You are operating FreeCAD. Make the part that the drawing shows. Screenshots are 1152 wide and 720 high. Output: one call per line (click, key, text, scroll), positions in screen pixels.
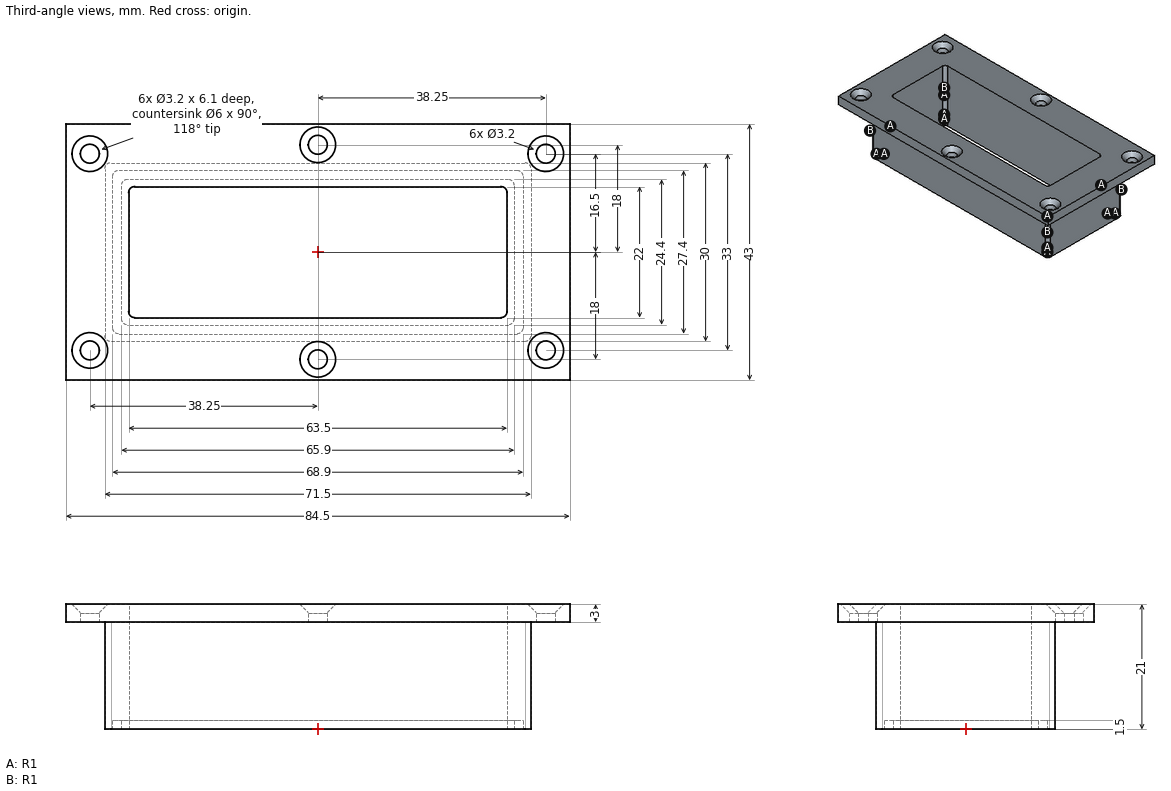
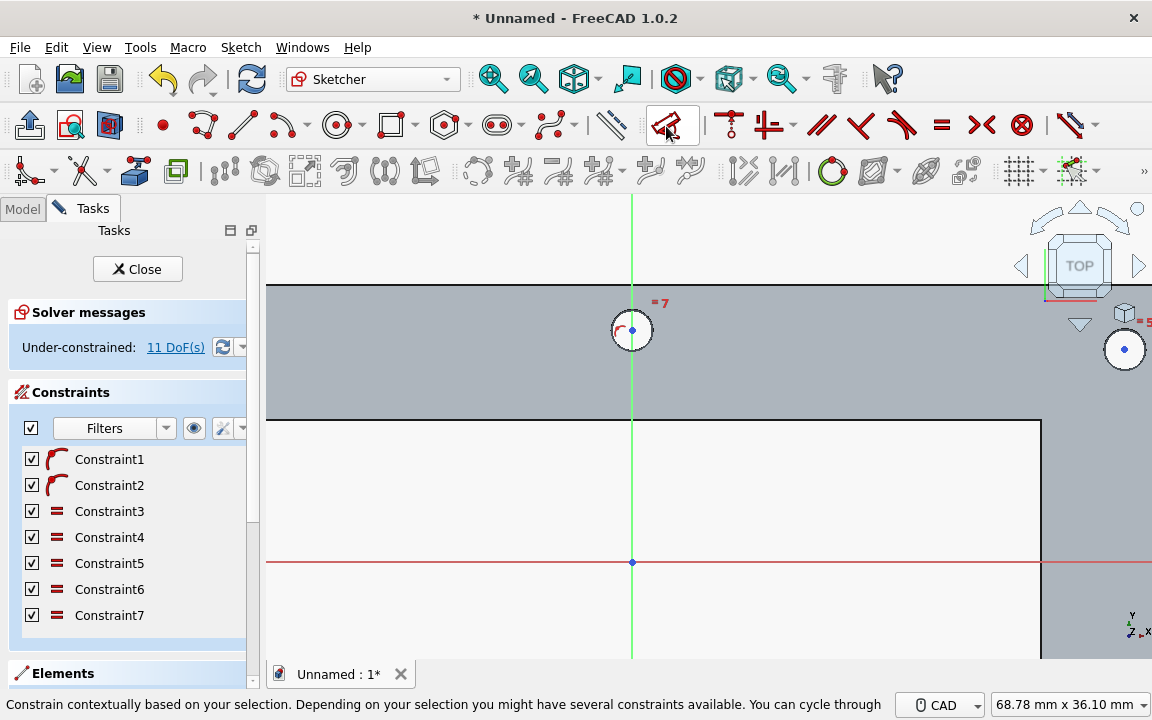
scroll(647, 316, down, 4)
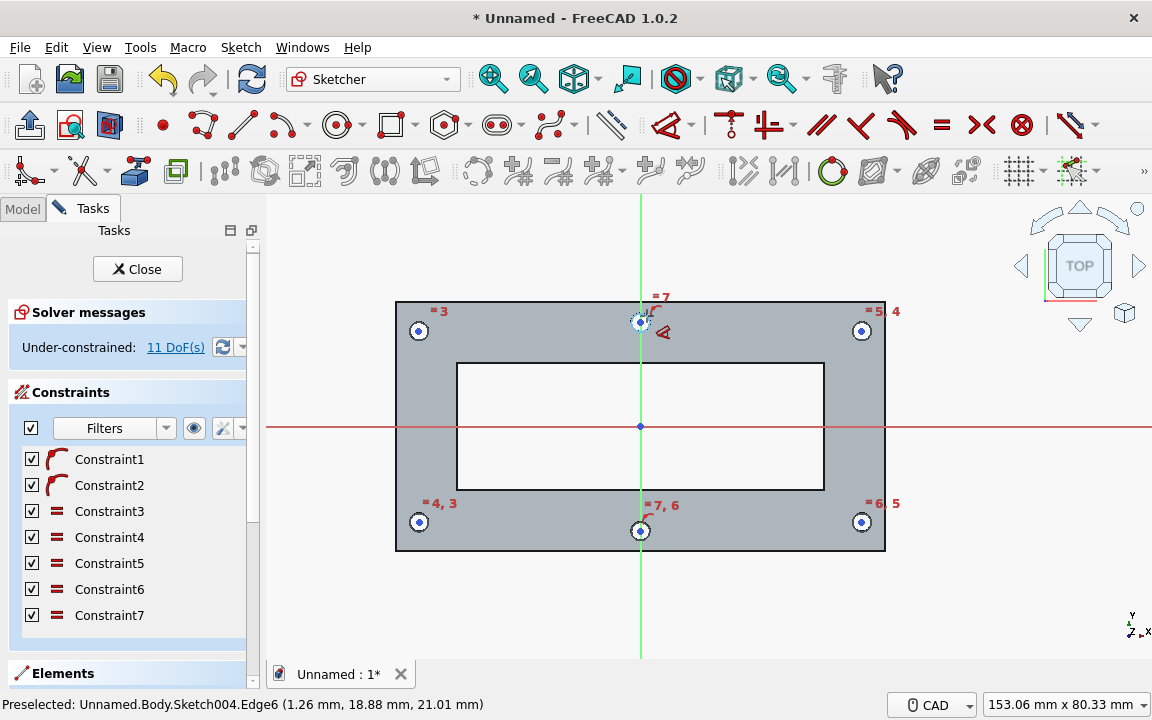
scroll(425, 325, up, 4)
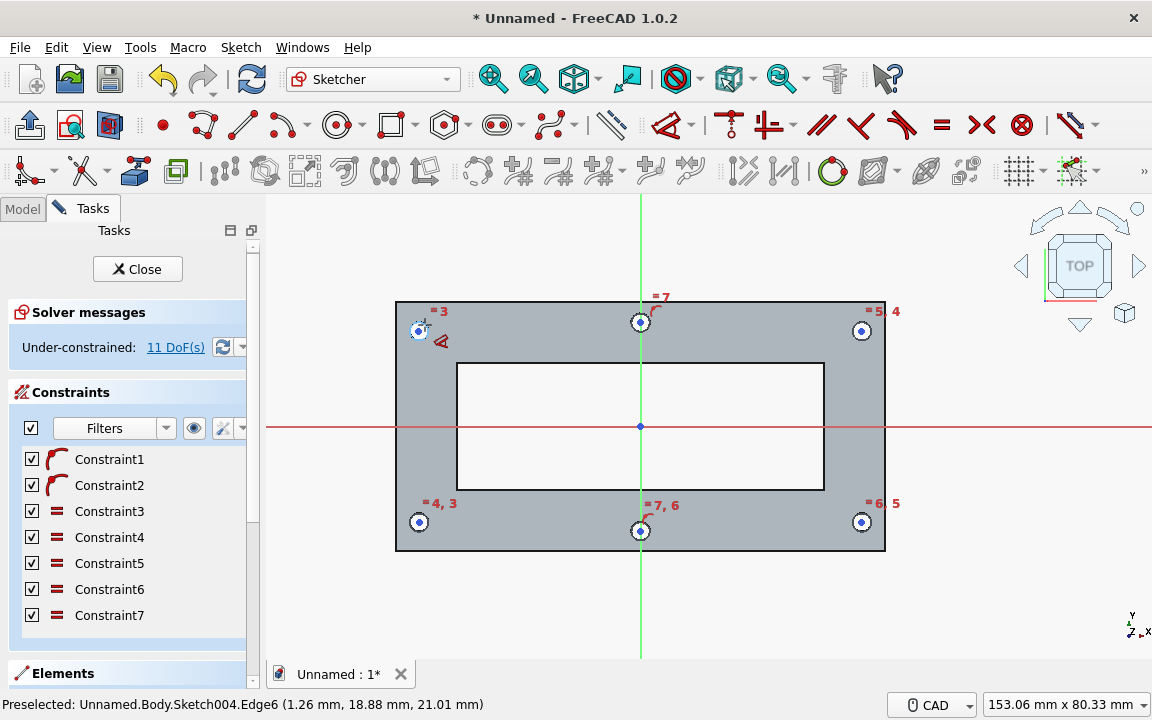
click(426, 325)
click(449, 303)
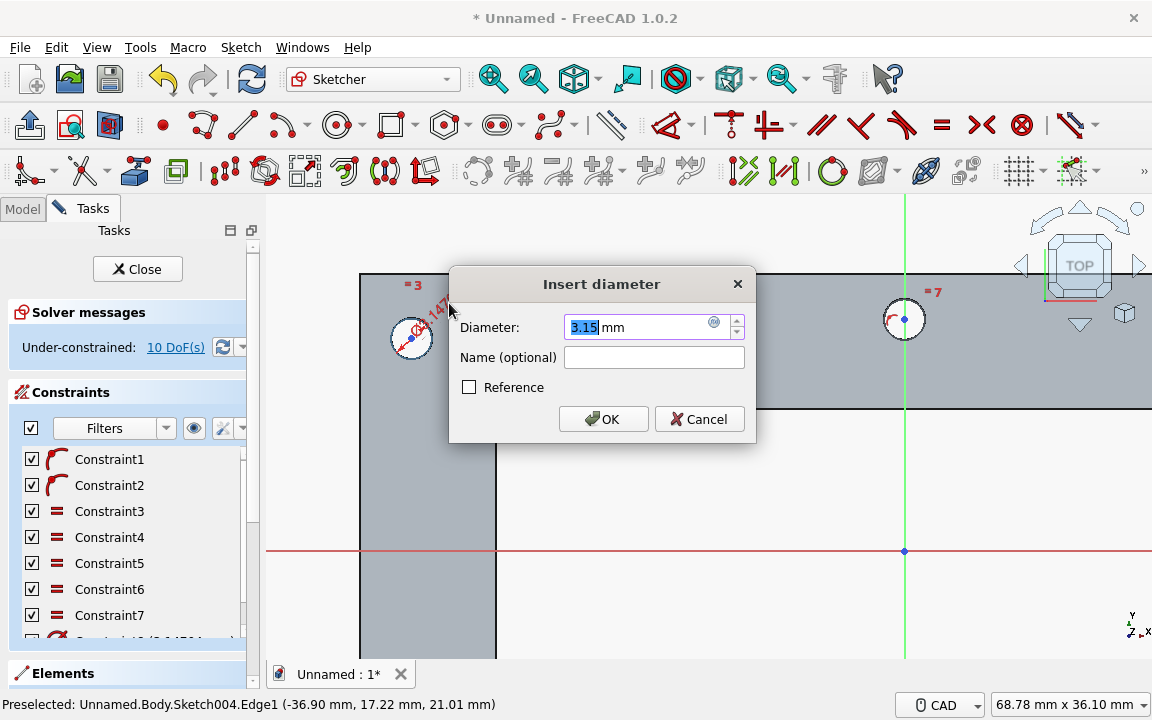
text(3.2)
key(Return)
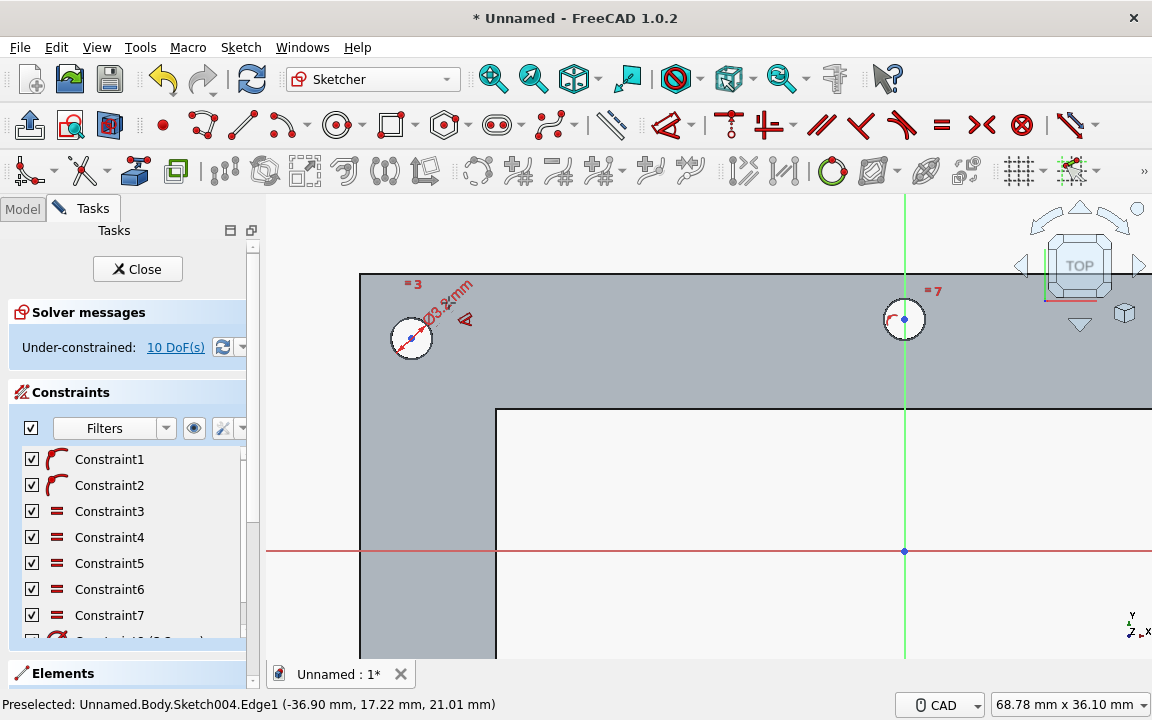
scroll(425, 325, down, 4)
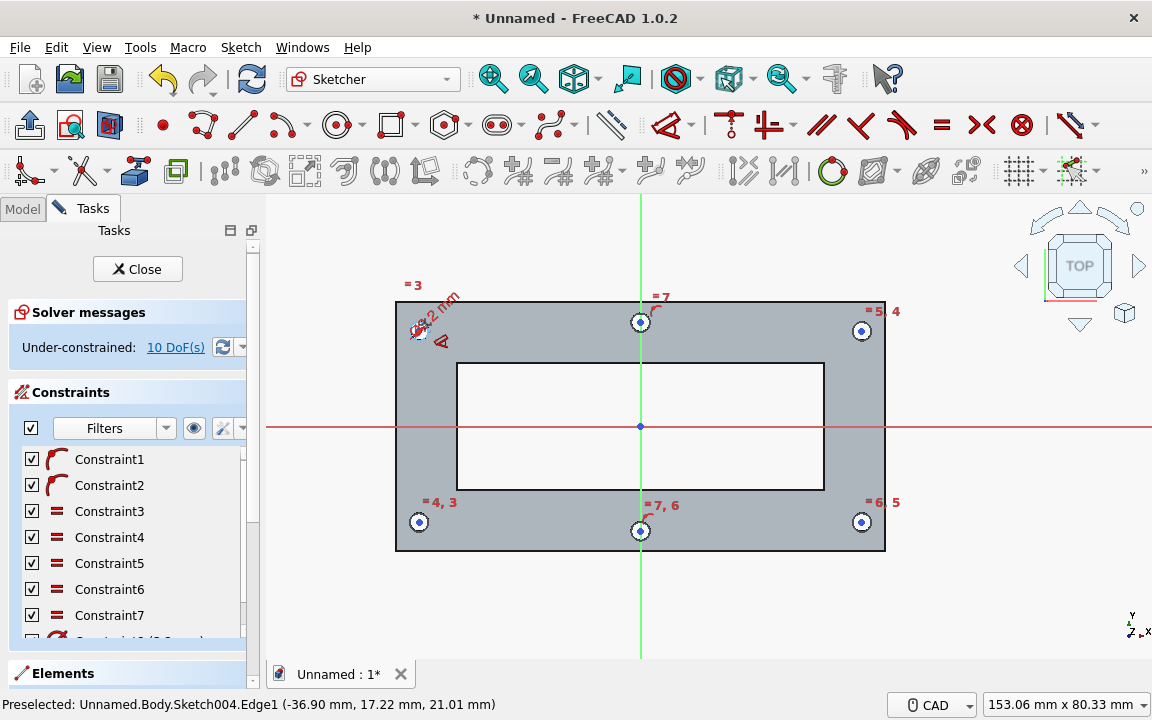
click(641, 531)
click(675, 479)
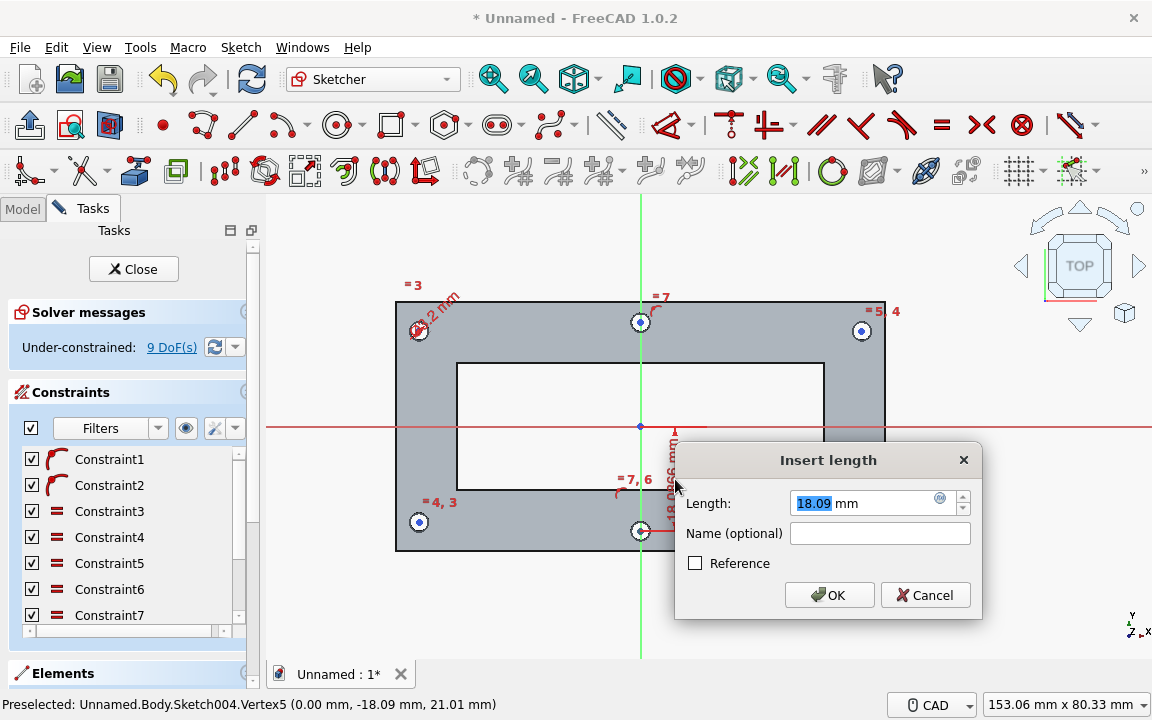
text(18)
key(Return)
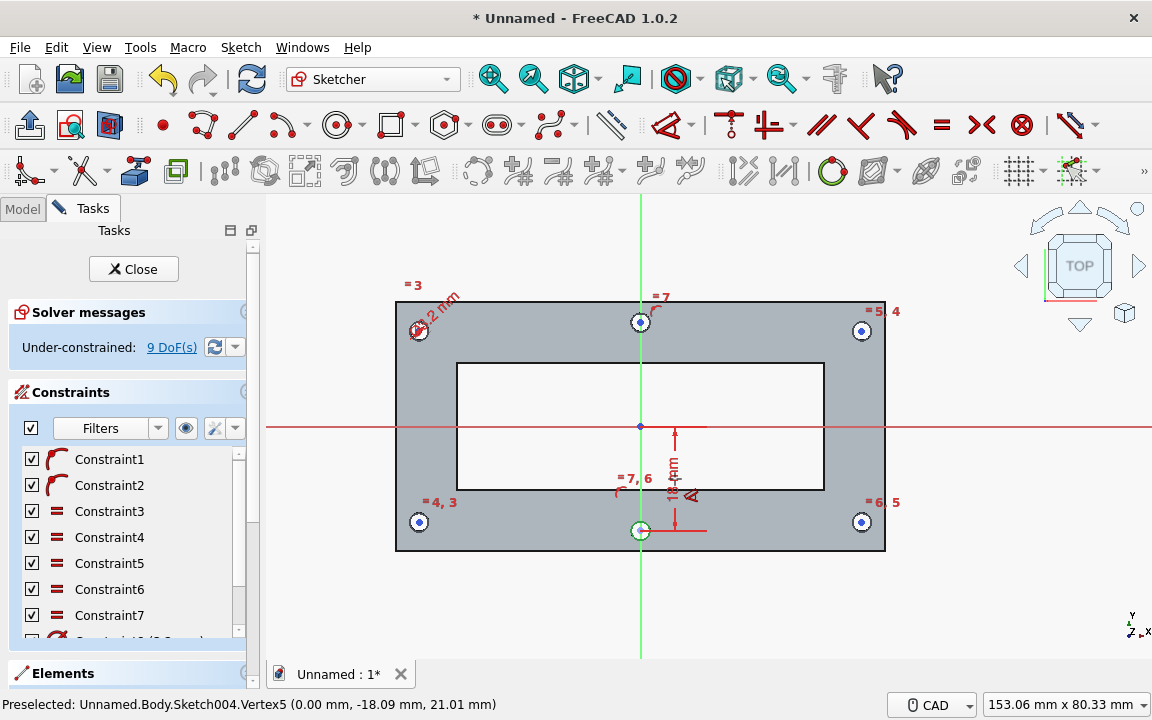
click(641, 323)
click(675, 375)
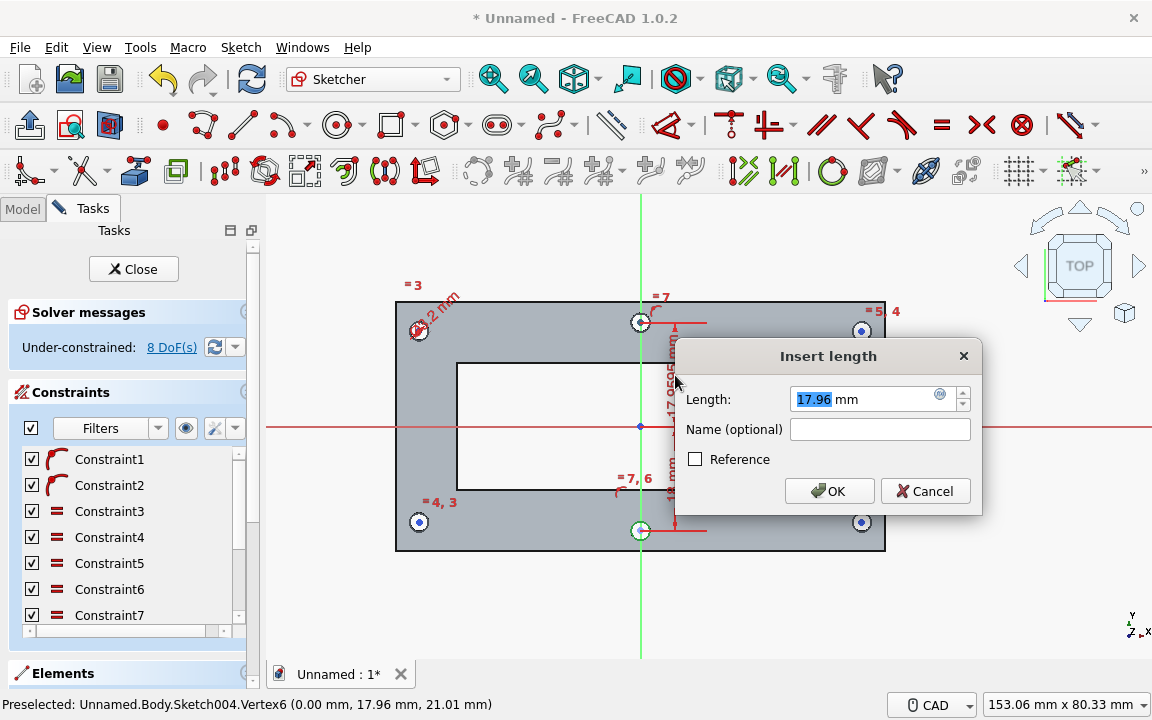
text(18)
key(Return)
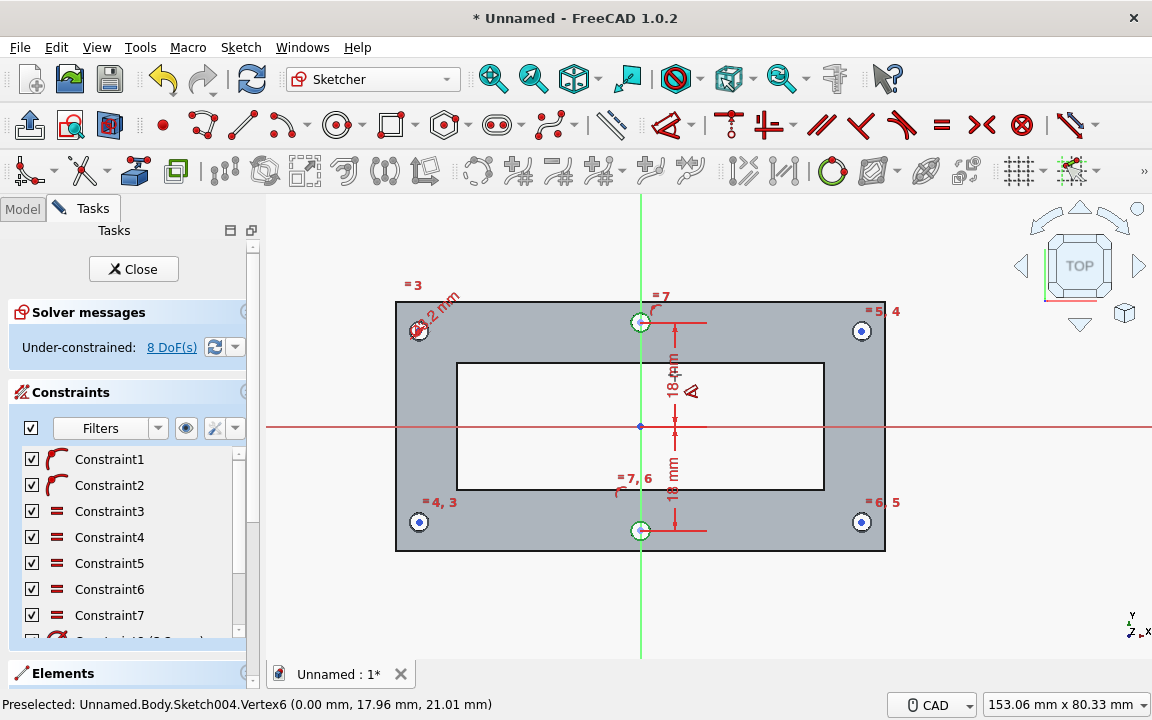
click(419, 331)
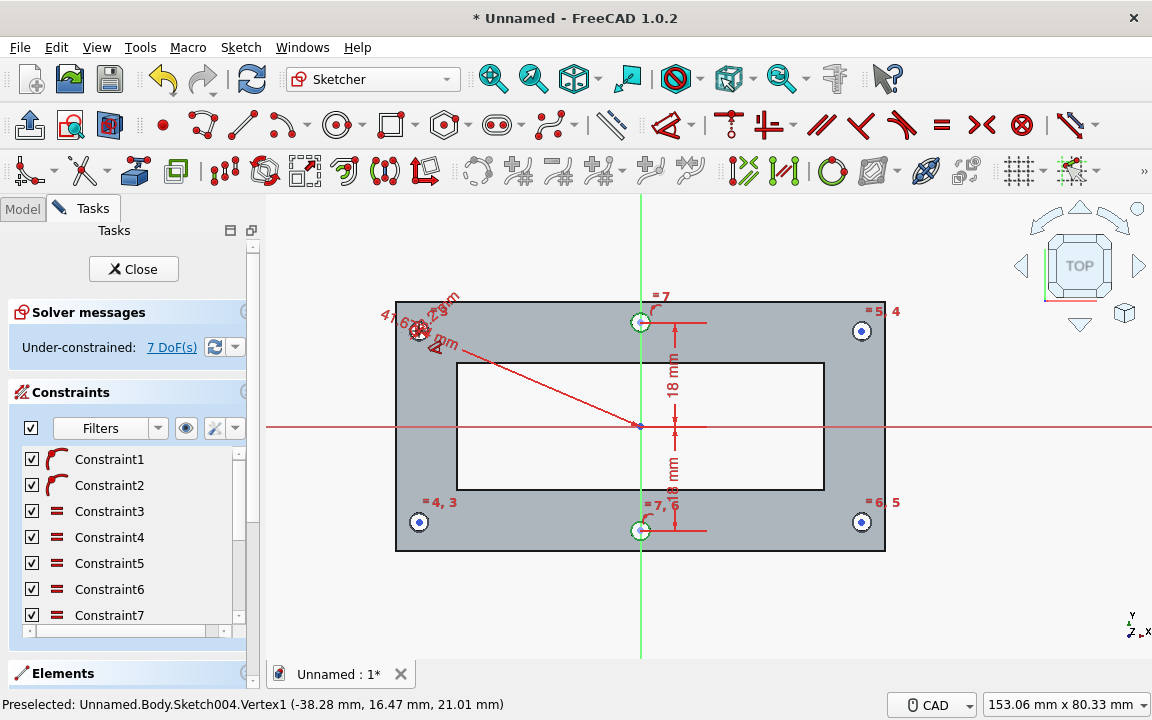
click(419, 523)
click(385, 383)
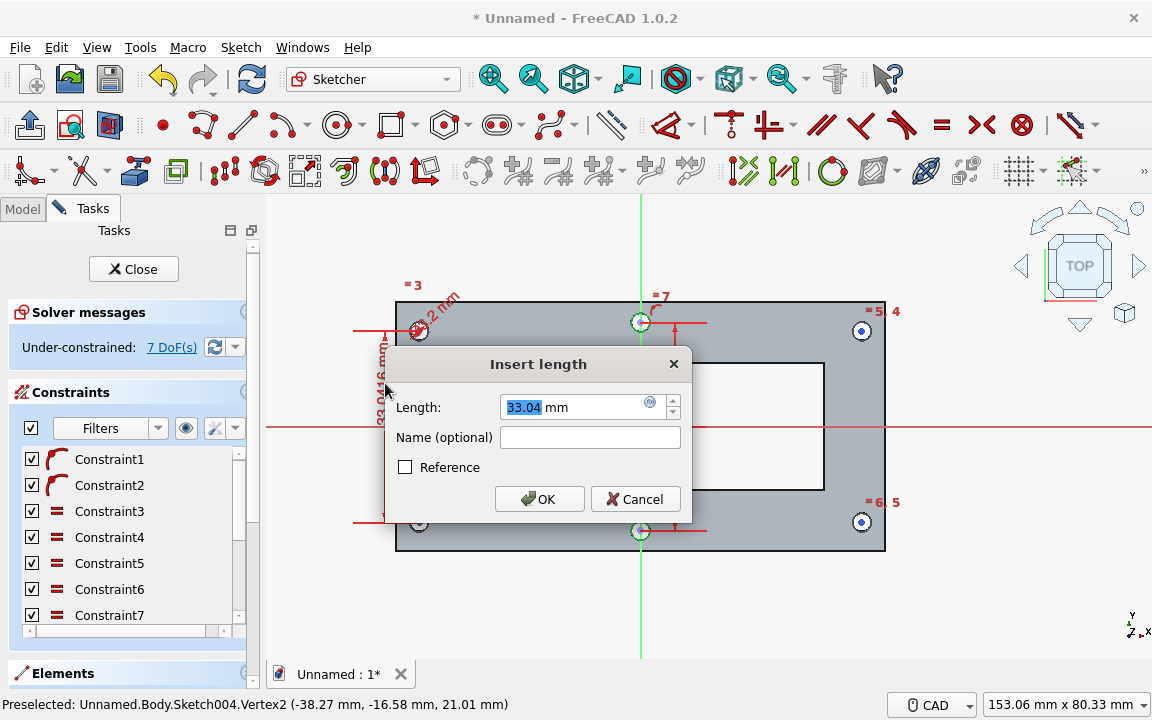
text(33)
key(Return)